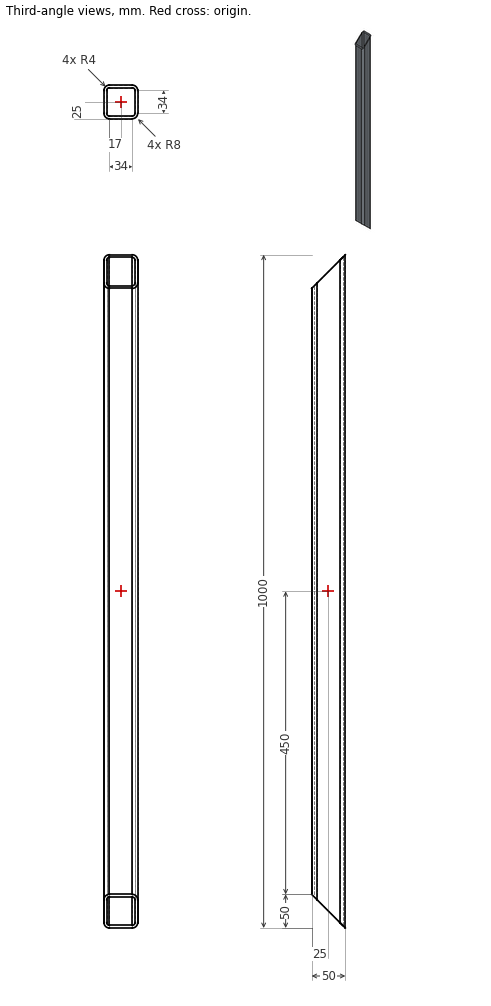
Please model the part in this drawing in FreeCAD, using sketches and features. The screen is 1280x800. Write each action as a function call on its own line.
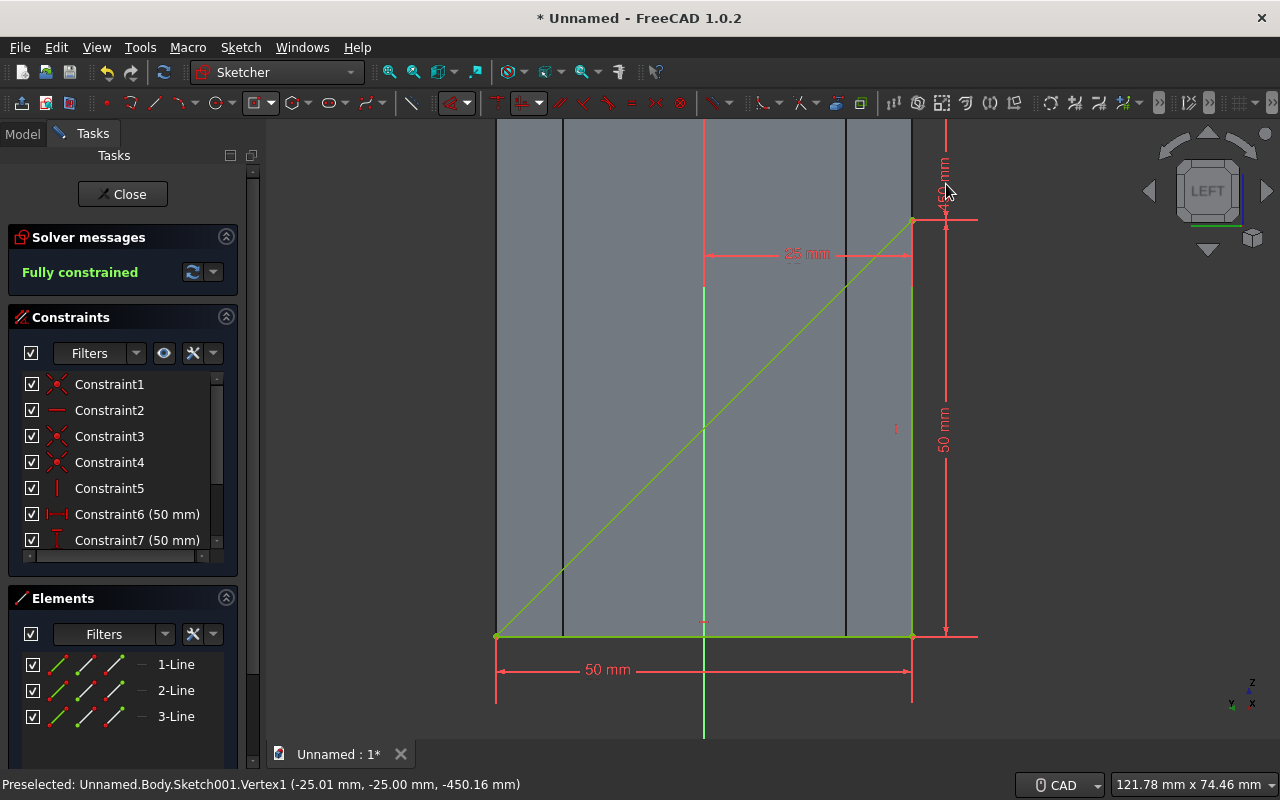
click(123, 194)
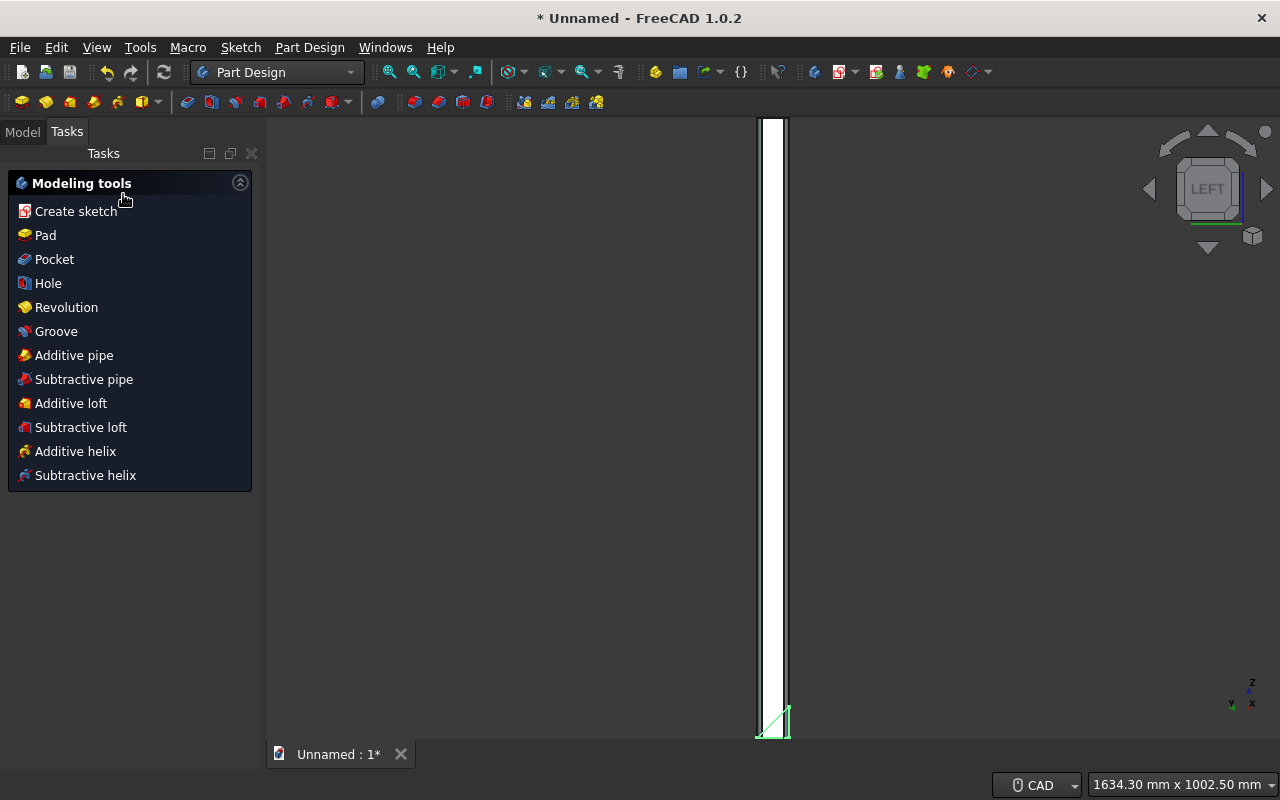
click(188, 102)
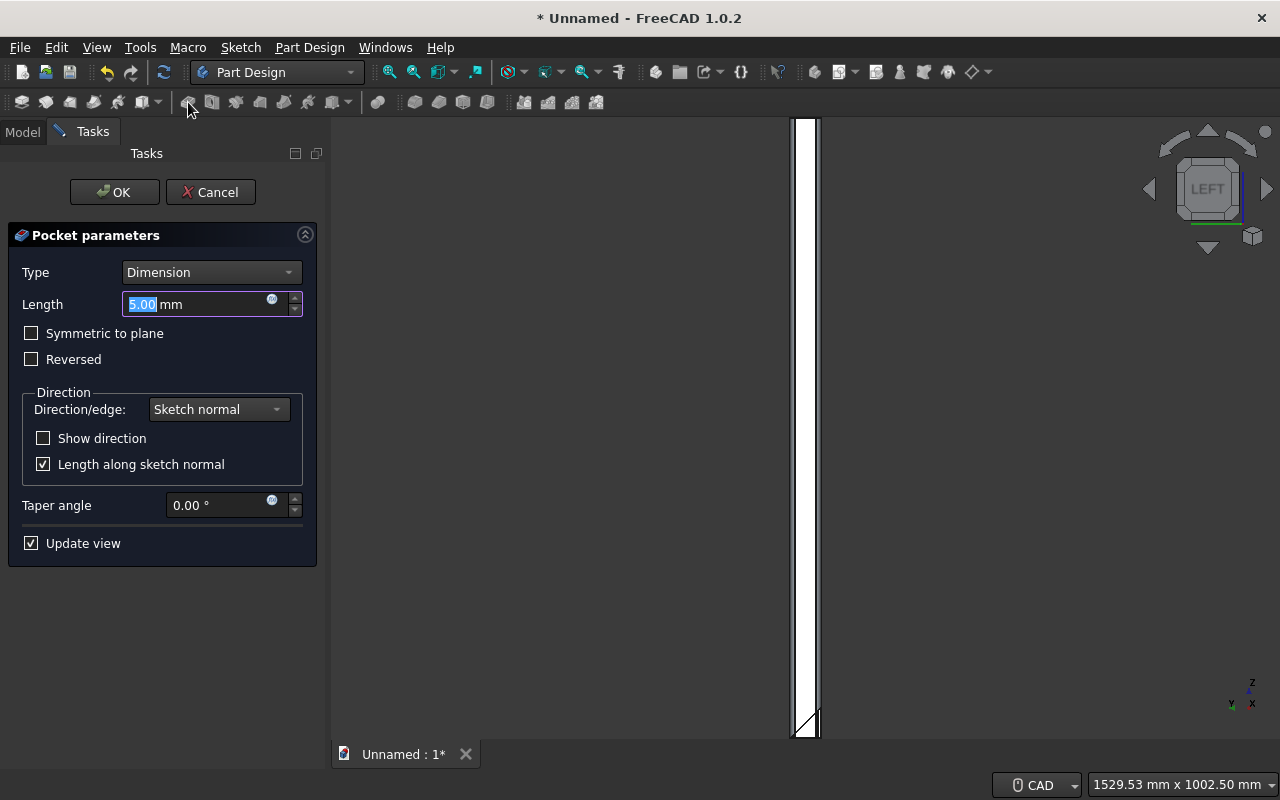
click(212, 272)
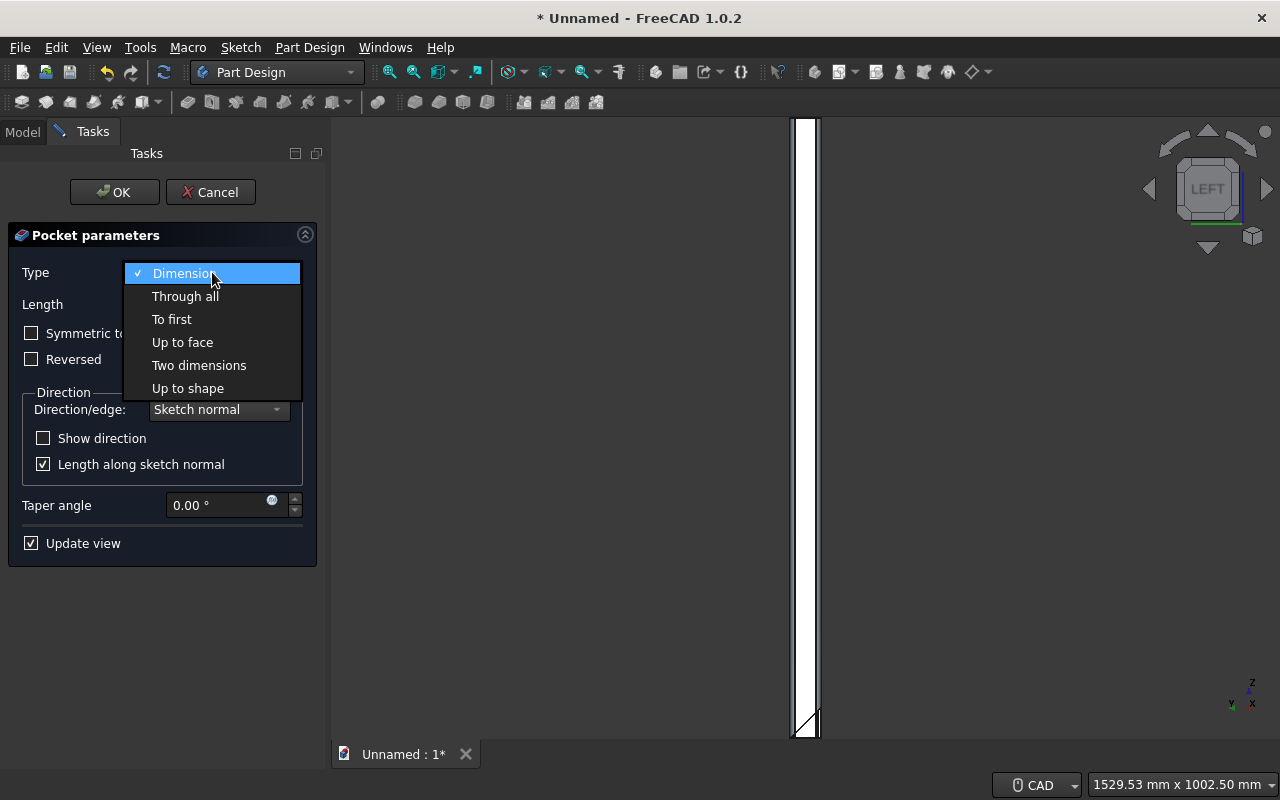
click(212, 296)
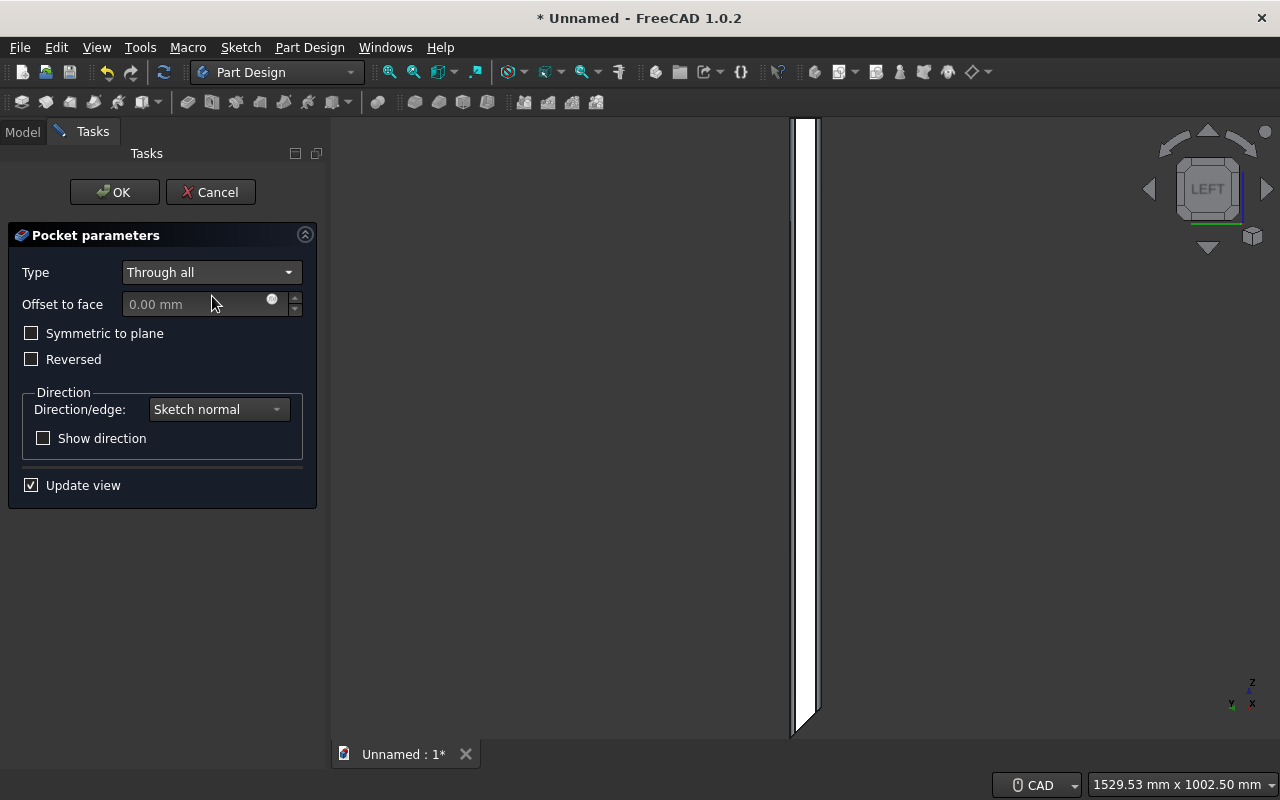
click(115, 192)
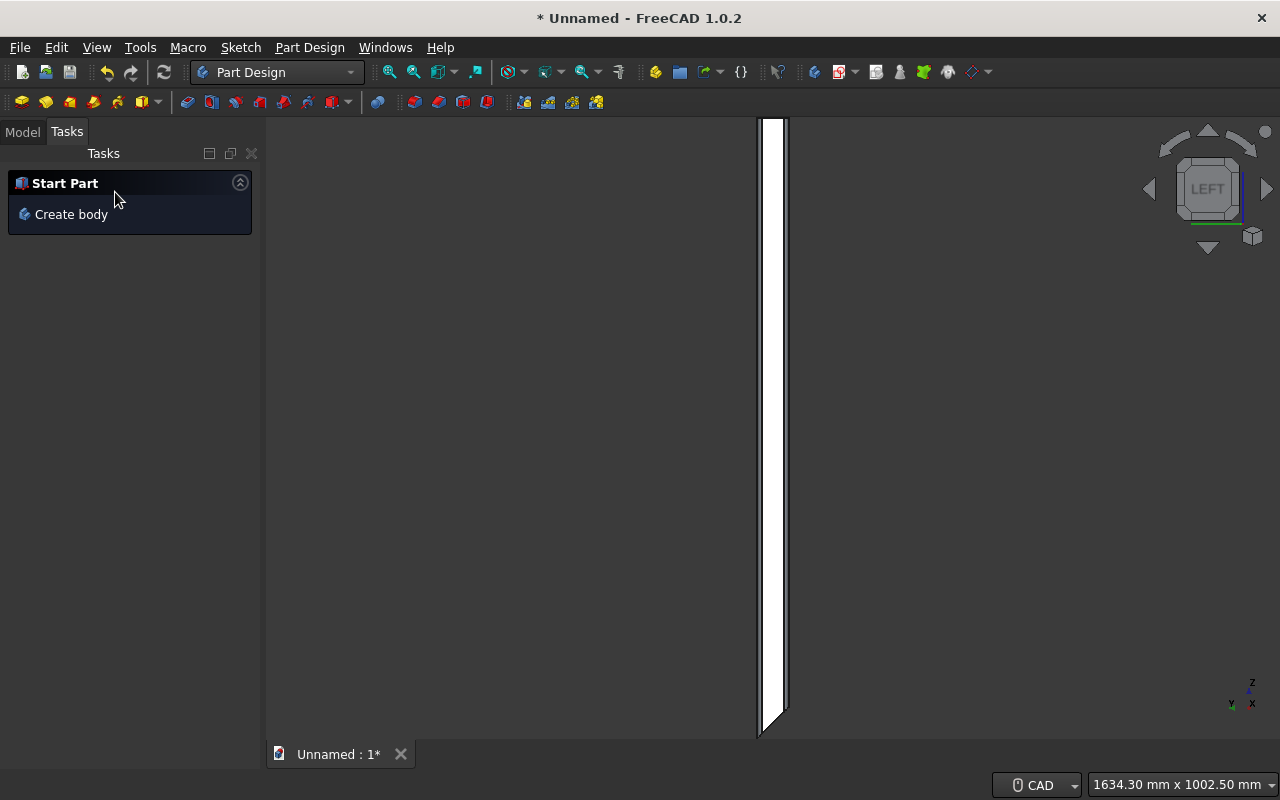
click(23, 131)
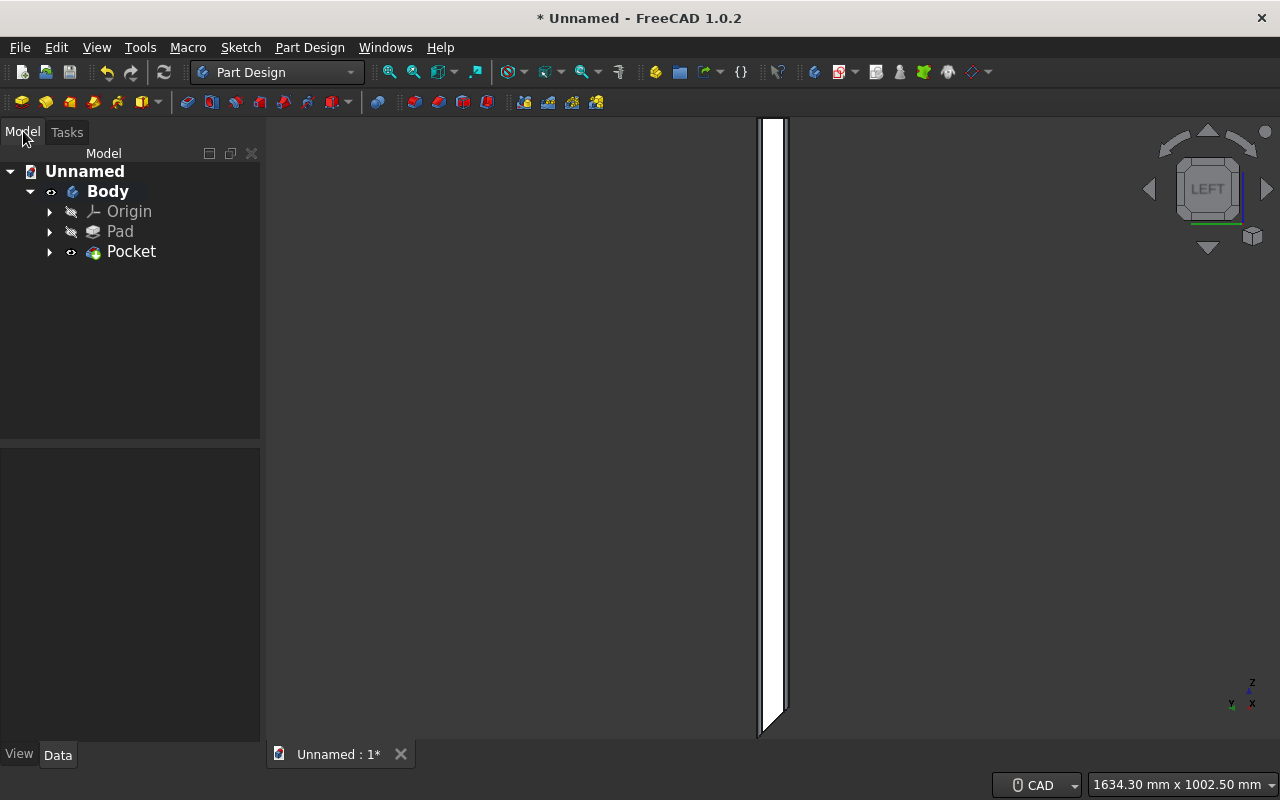
click(116, 252)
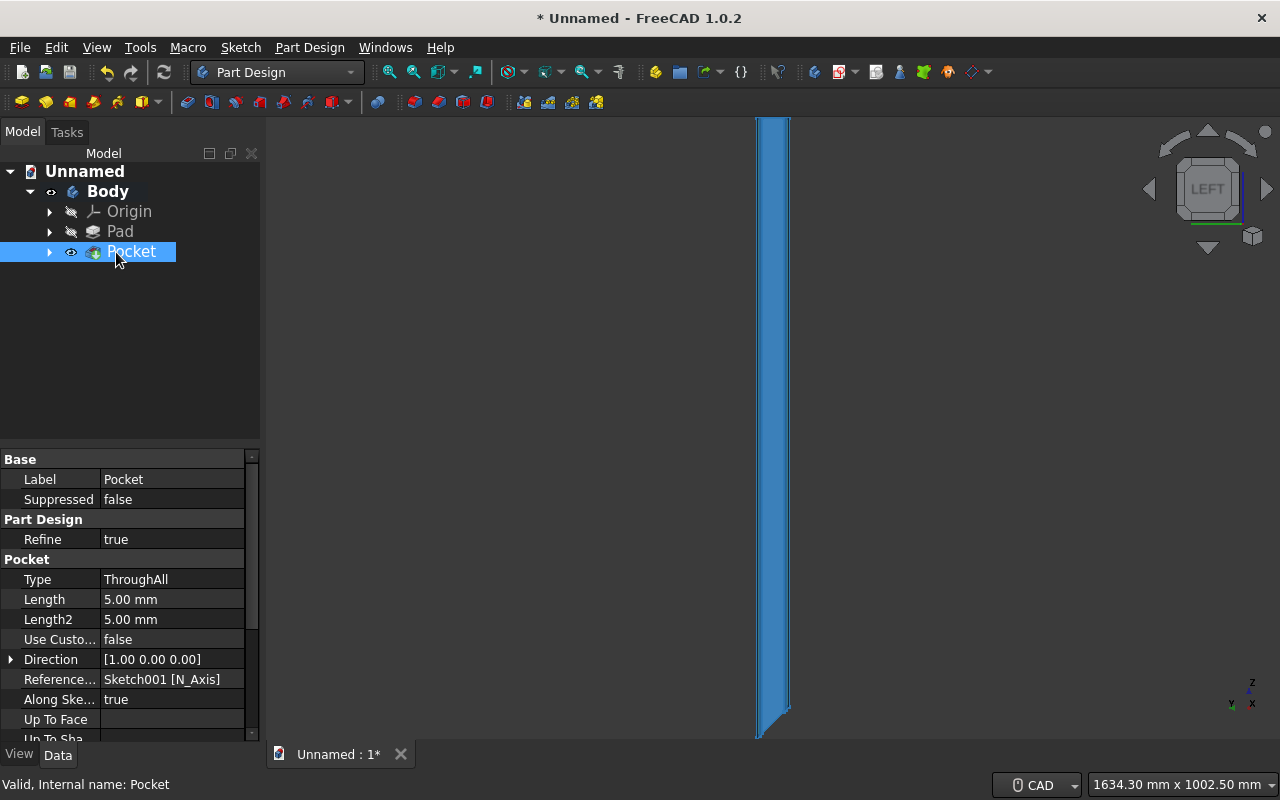
click(524, 102)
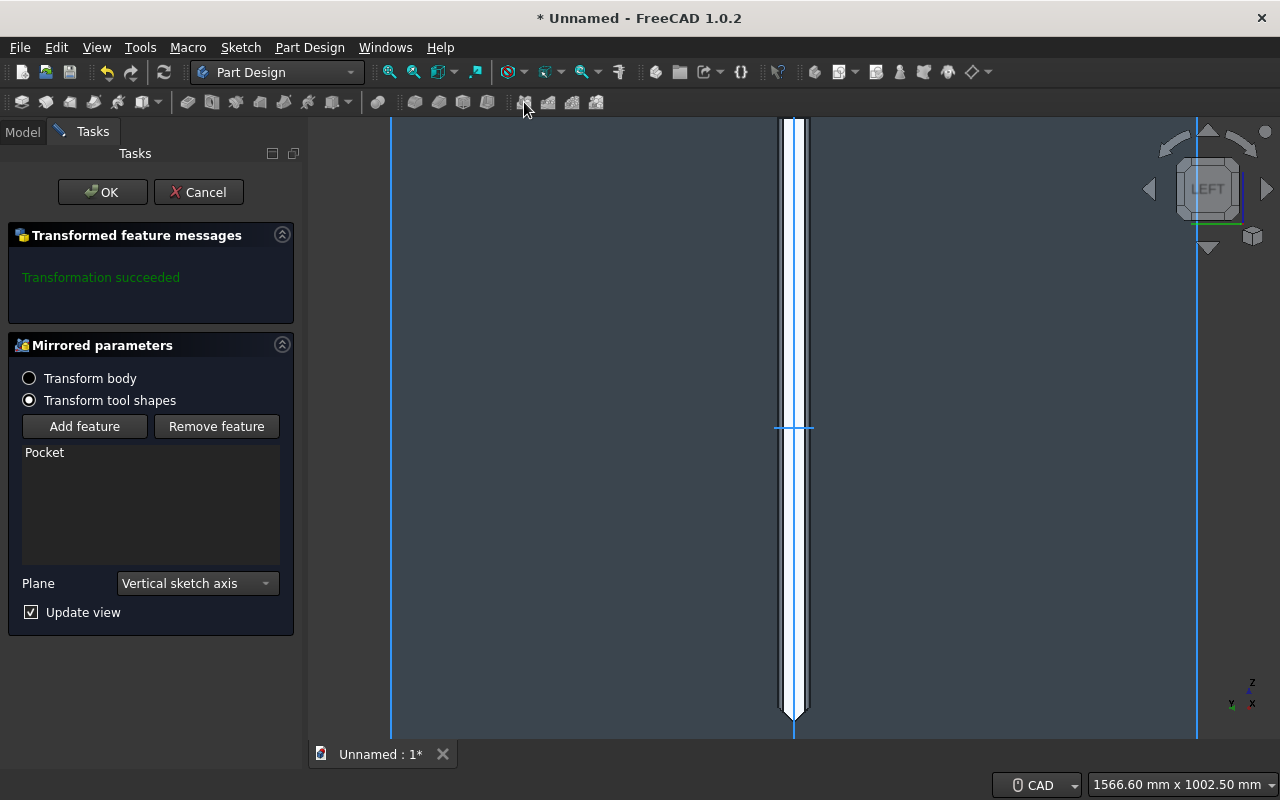
click(198, 584)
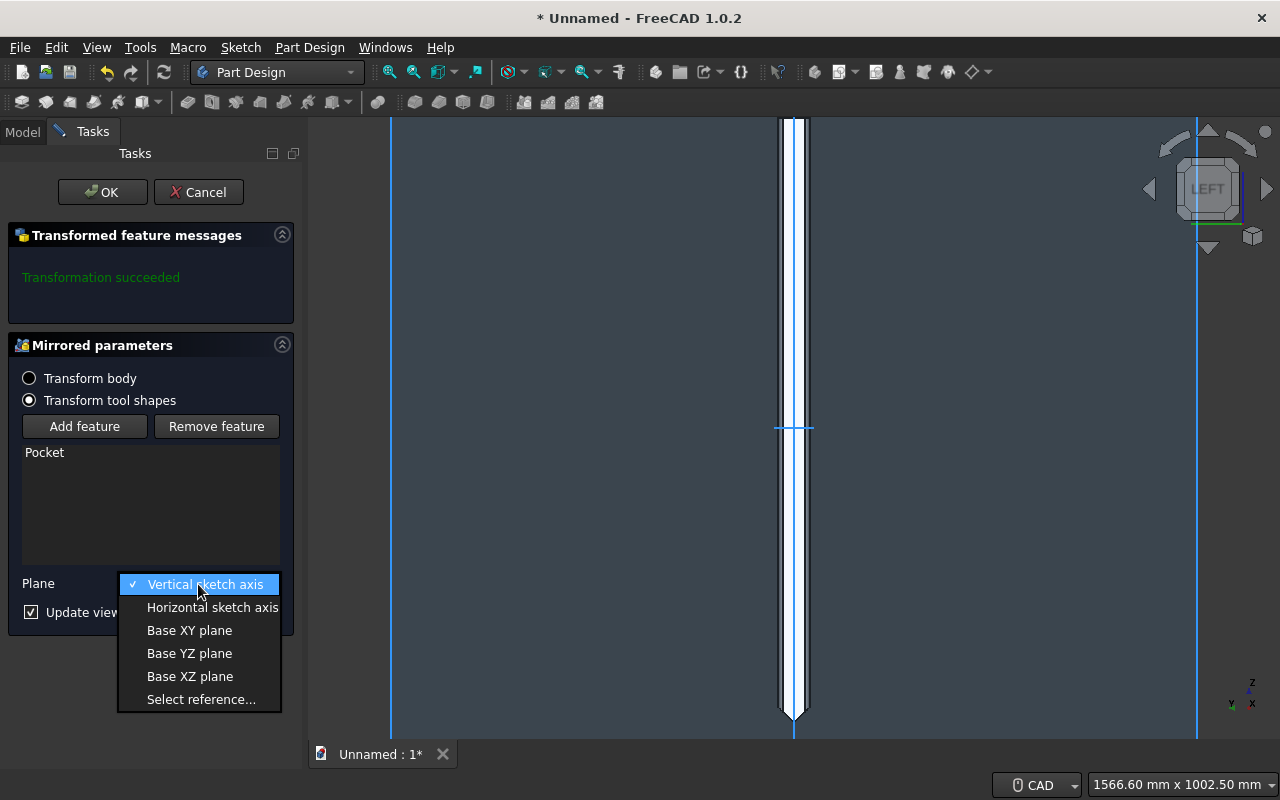
click(198, 630)